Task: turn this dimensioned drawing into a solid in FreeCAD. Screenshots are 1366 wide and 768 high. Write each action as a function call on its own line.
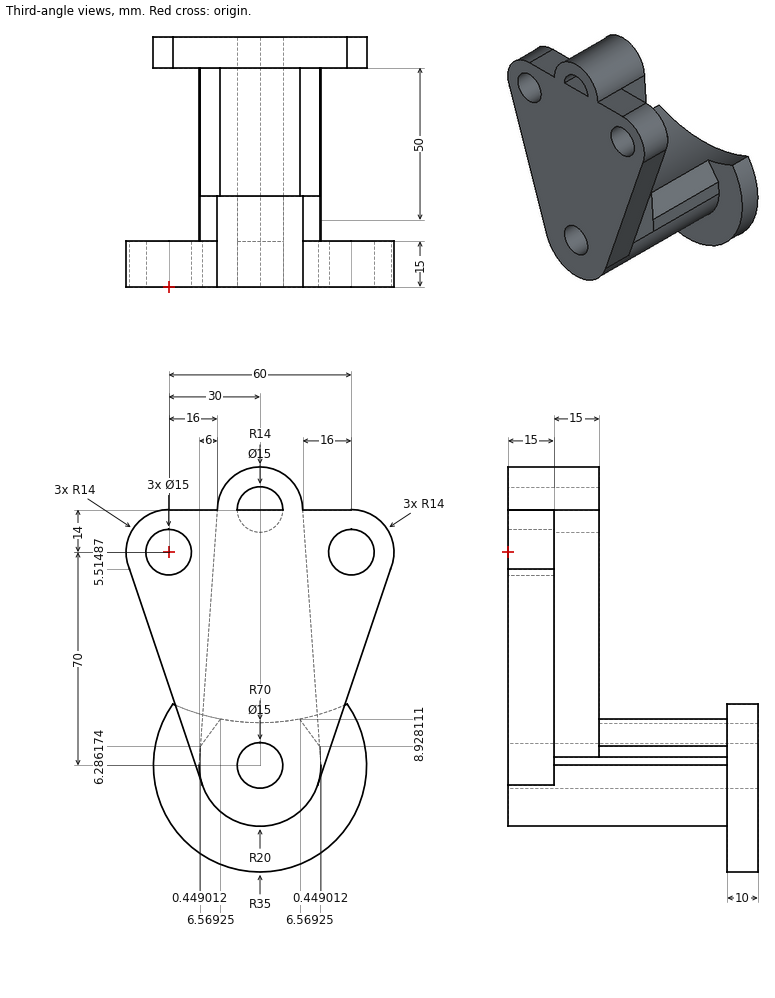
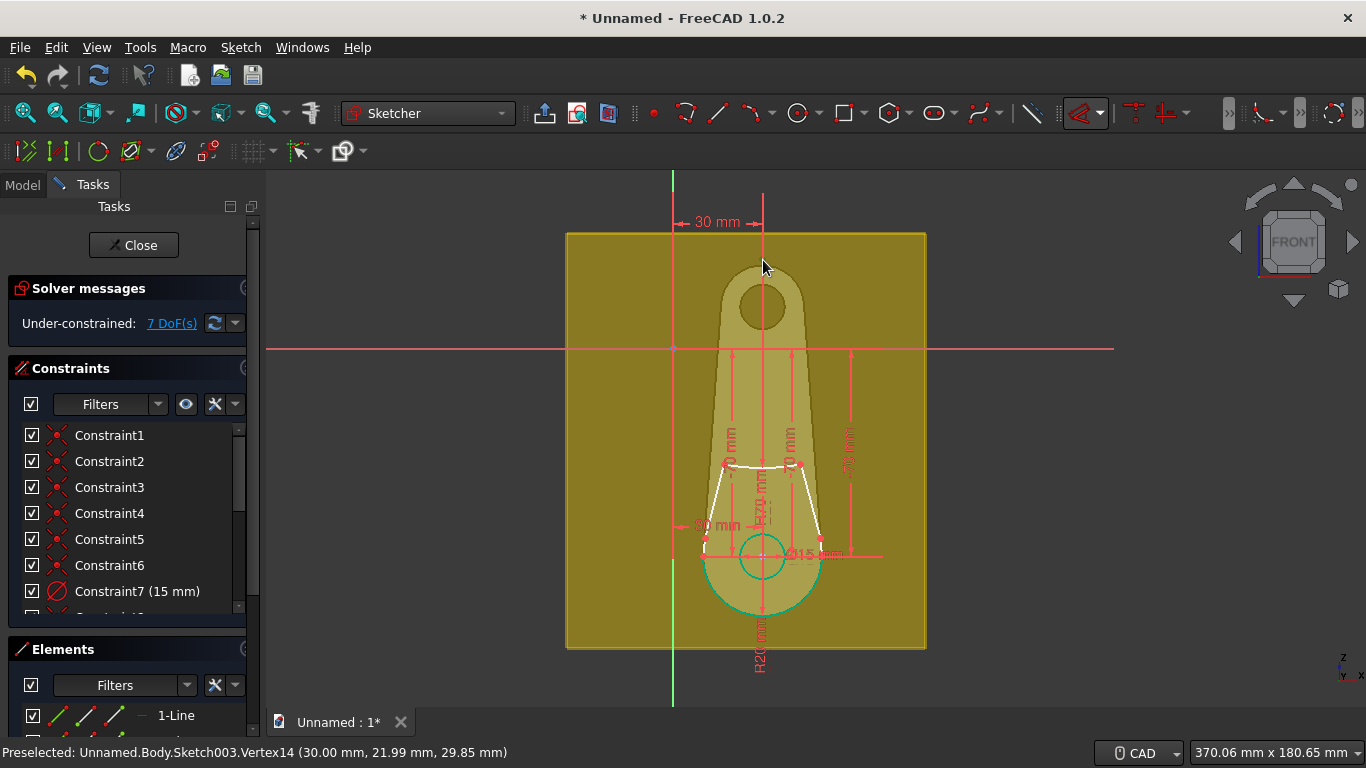
click(1102, 114)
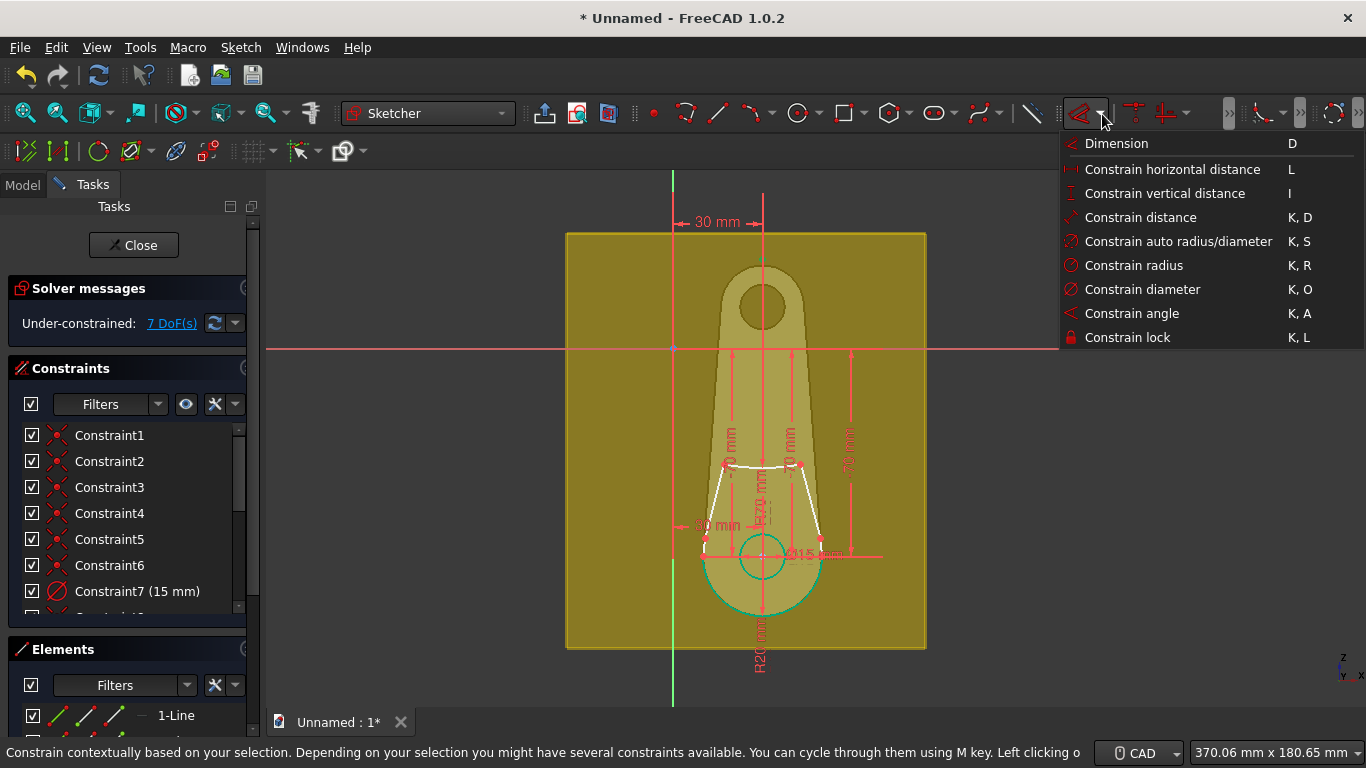
click(1212, 193)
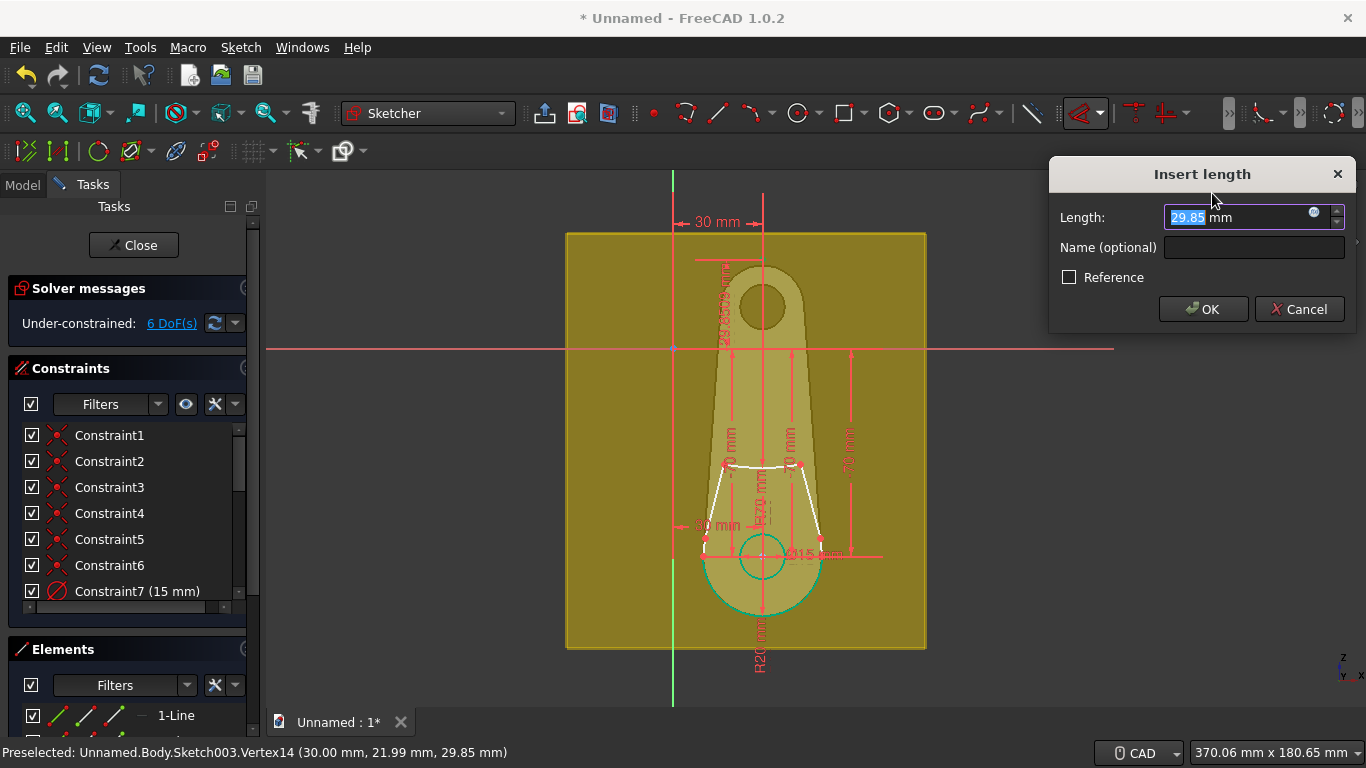
text(14)
key(Return)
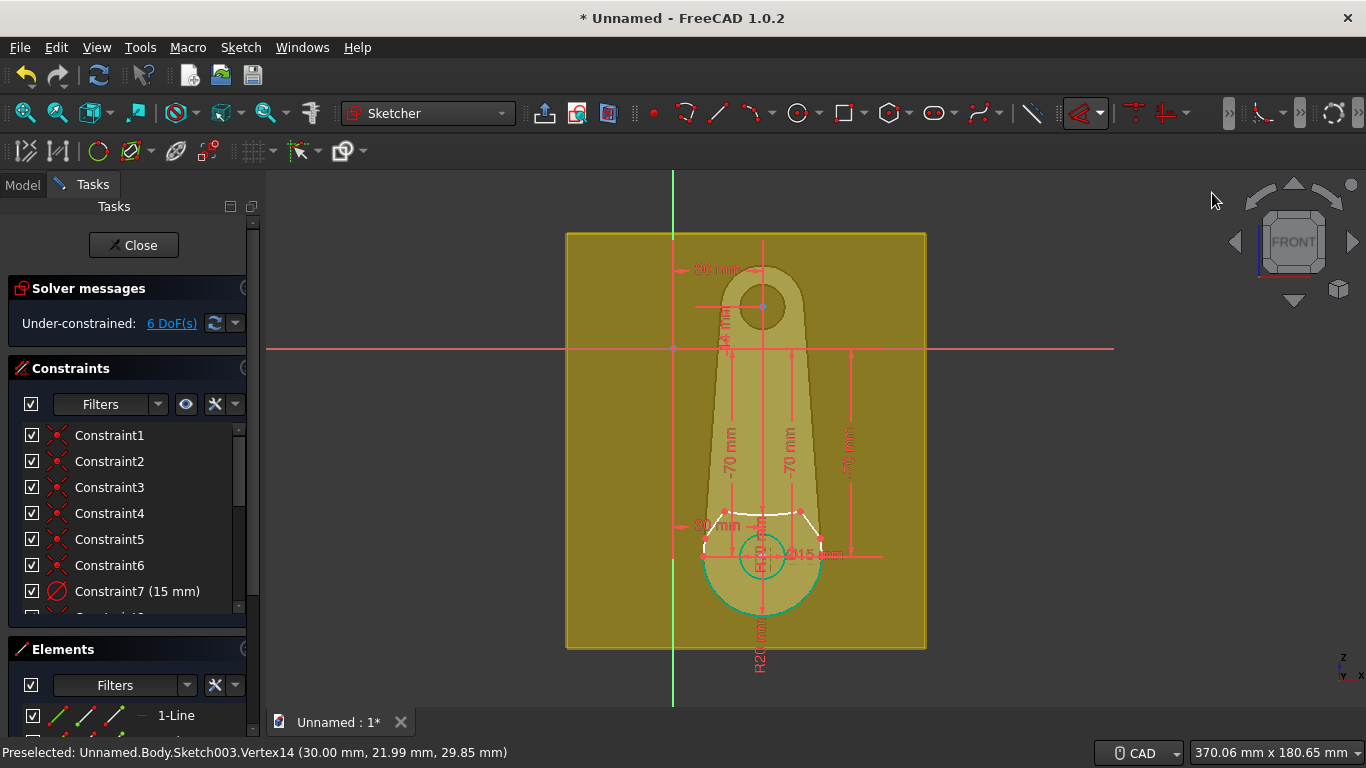
scroll(807, 520, up, 4)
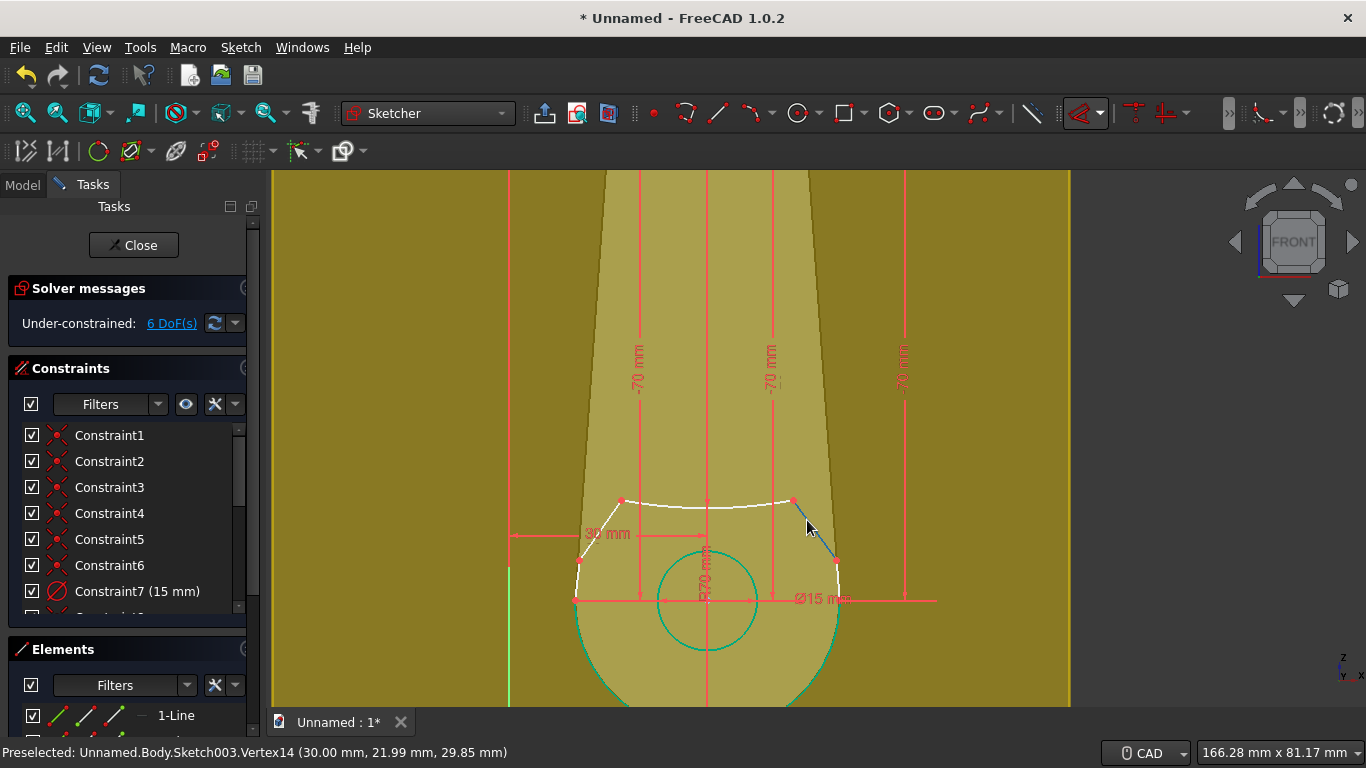
click(806, 518)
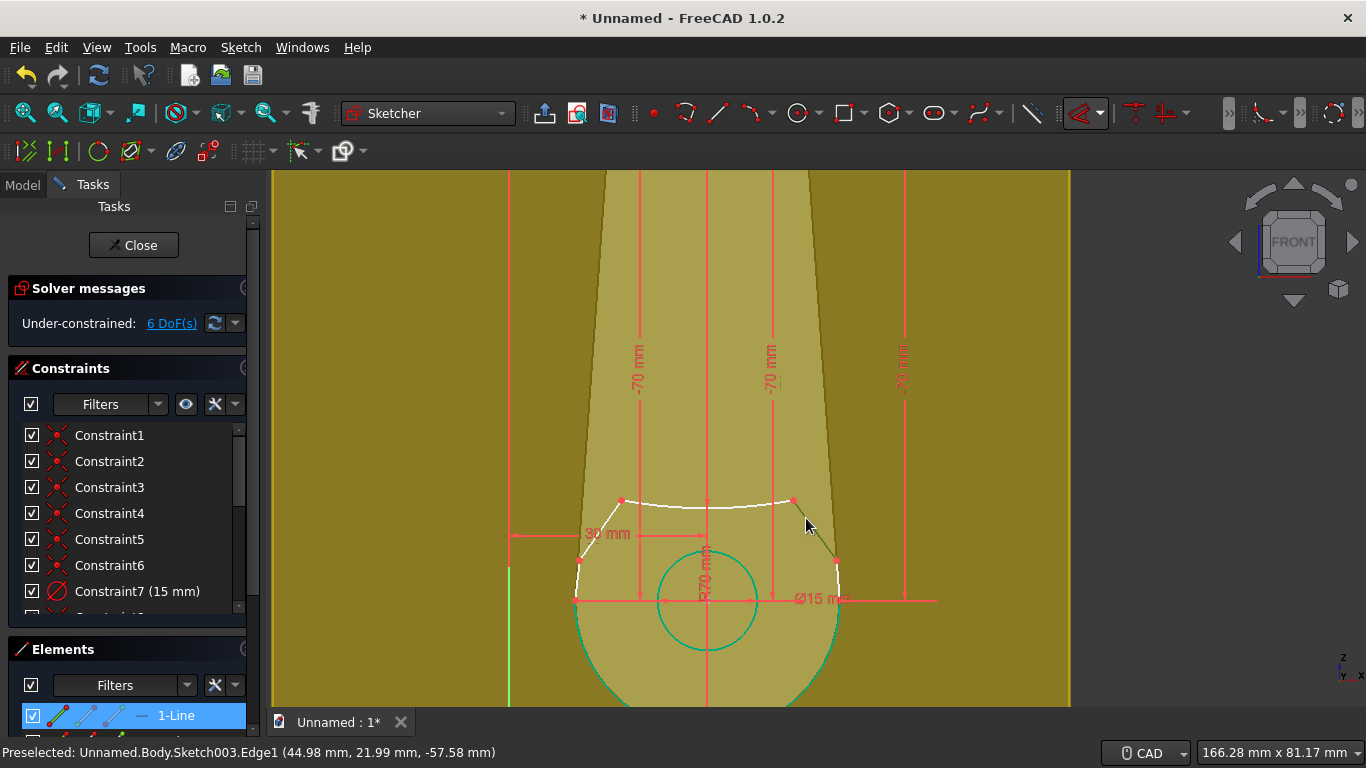
key(l)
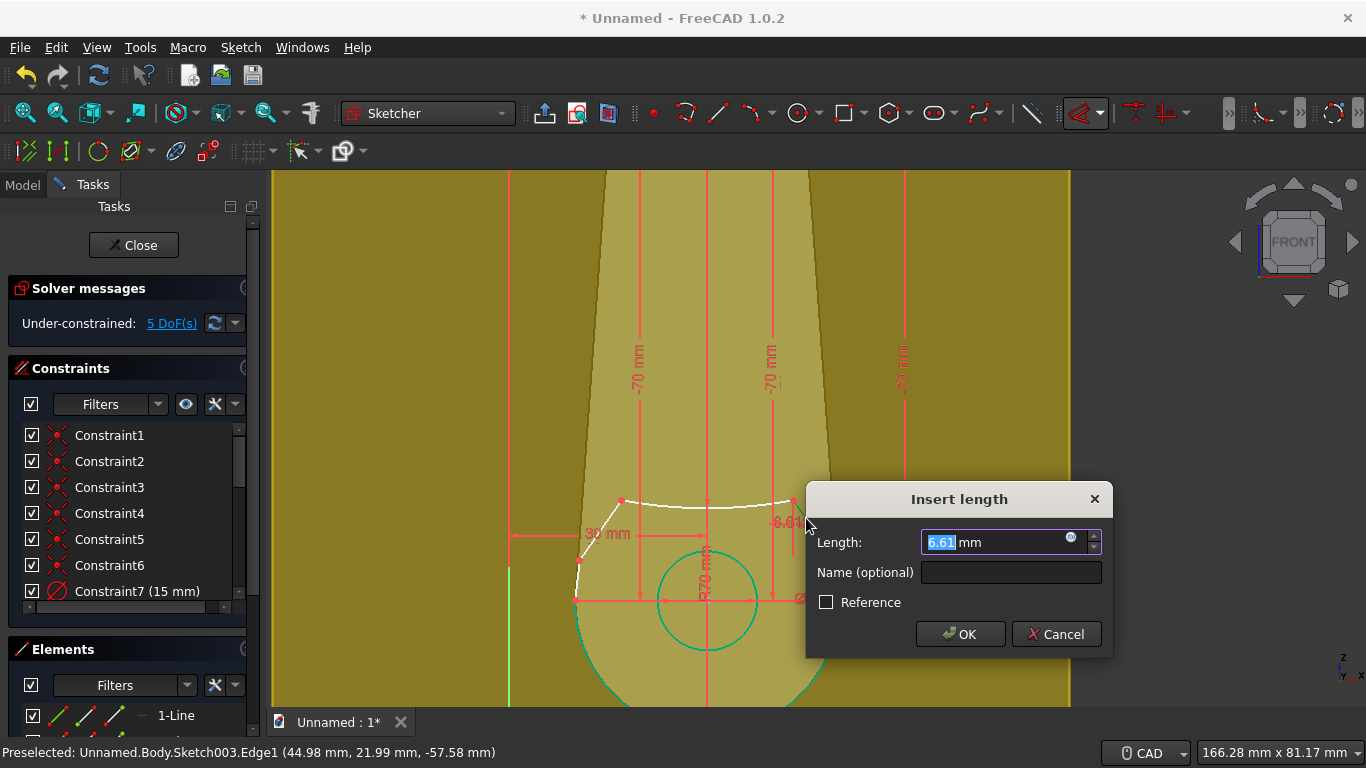
text(6.56925)
key(Return)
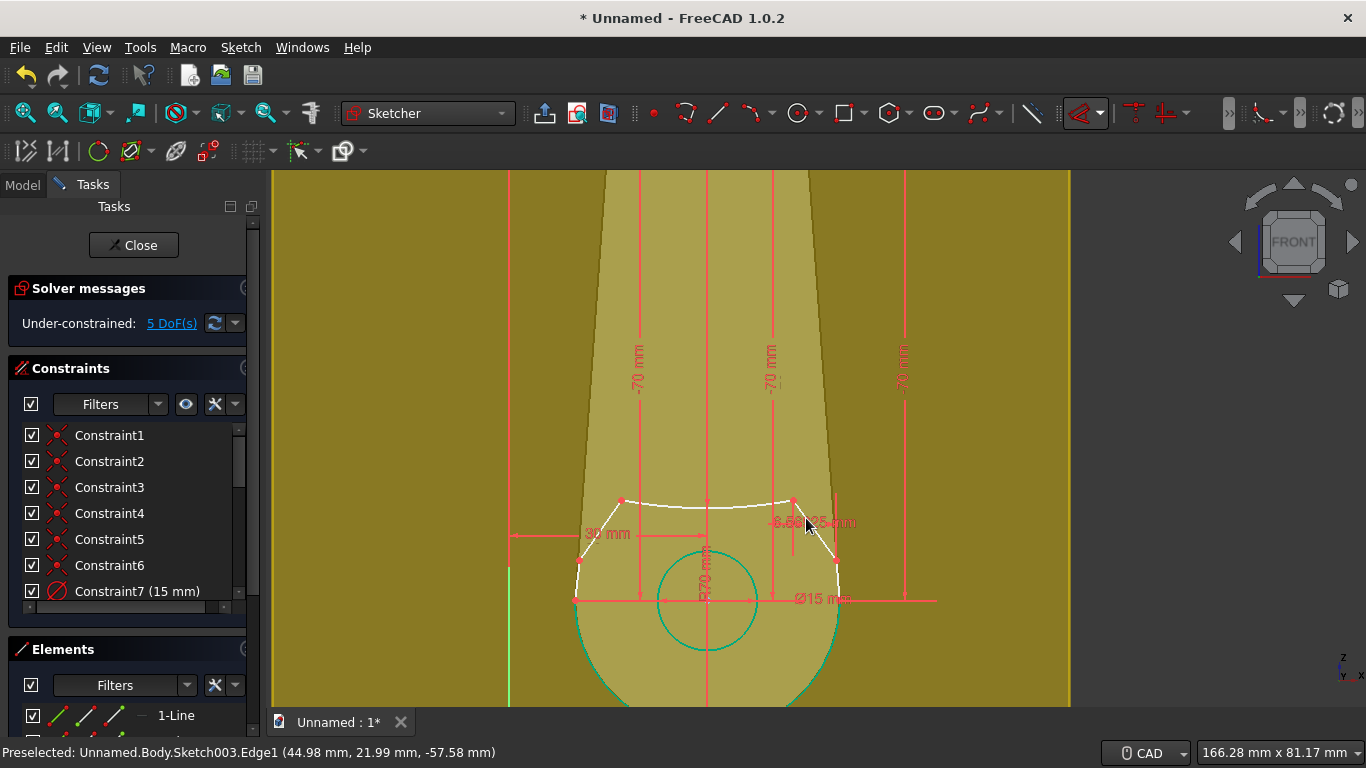
click(609, 518)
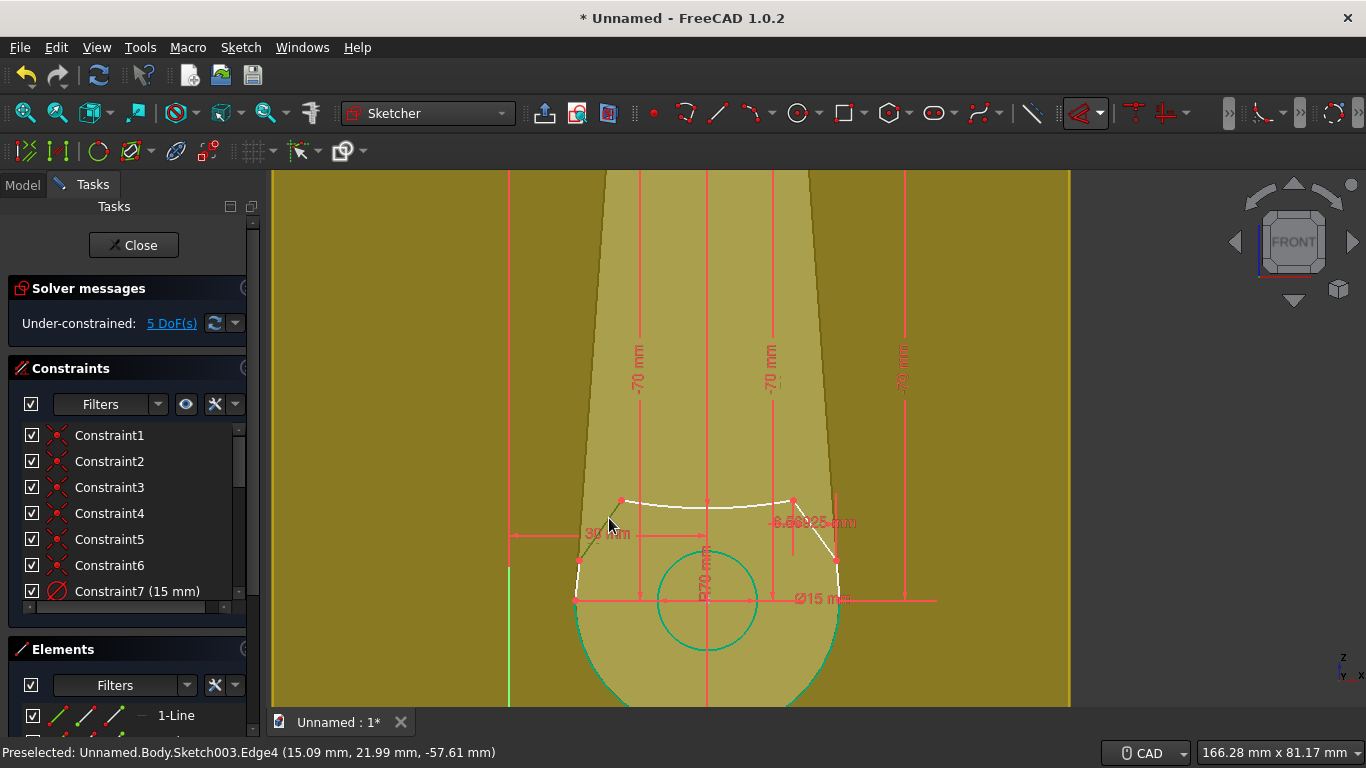
key(l)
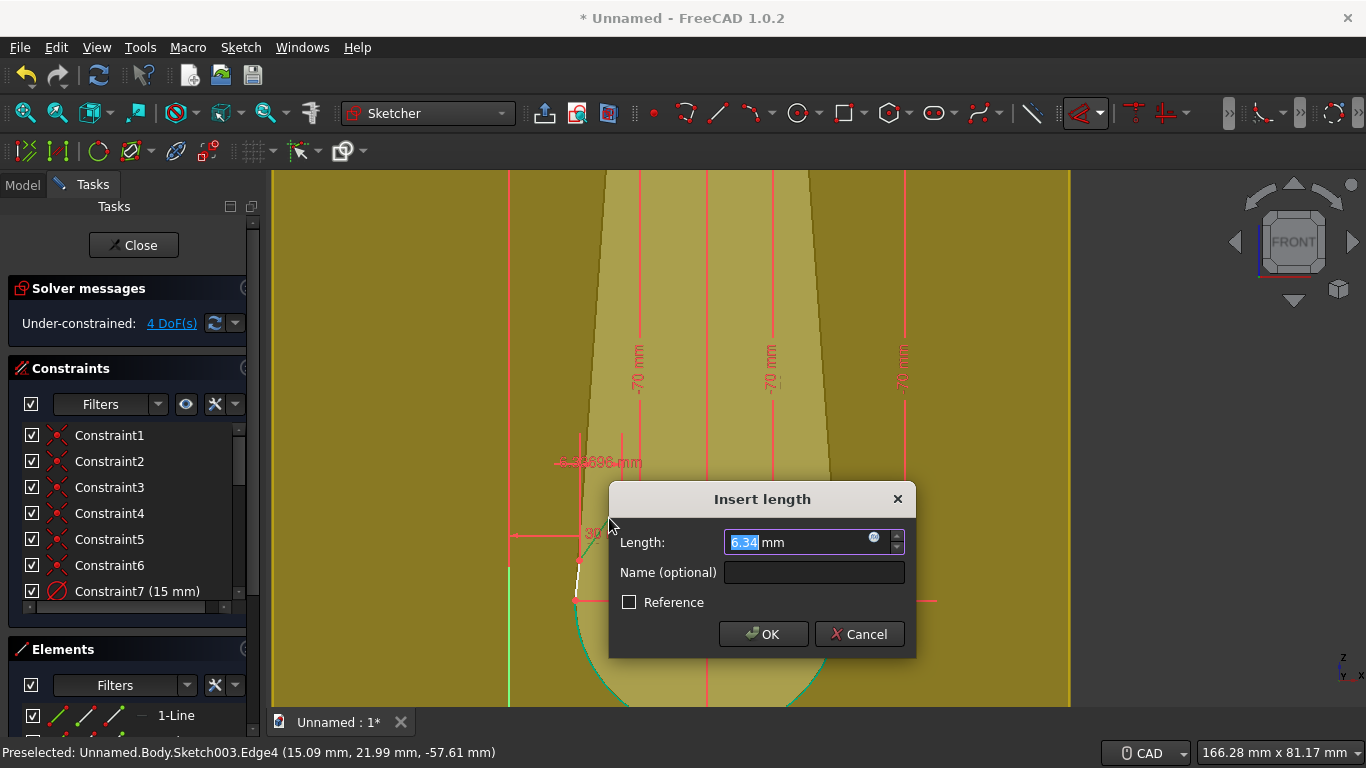
text(6.56925)
key(Return)